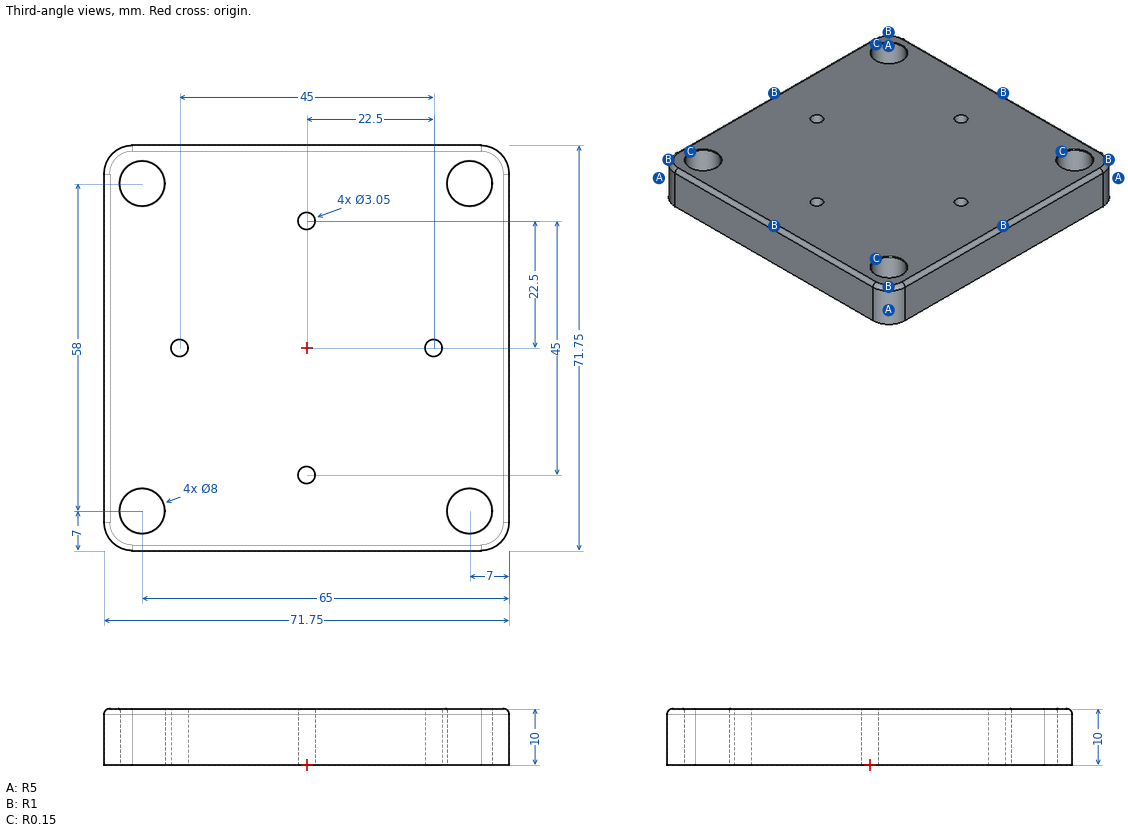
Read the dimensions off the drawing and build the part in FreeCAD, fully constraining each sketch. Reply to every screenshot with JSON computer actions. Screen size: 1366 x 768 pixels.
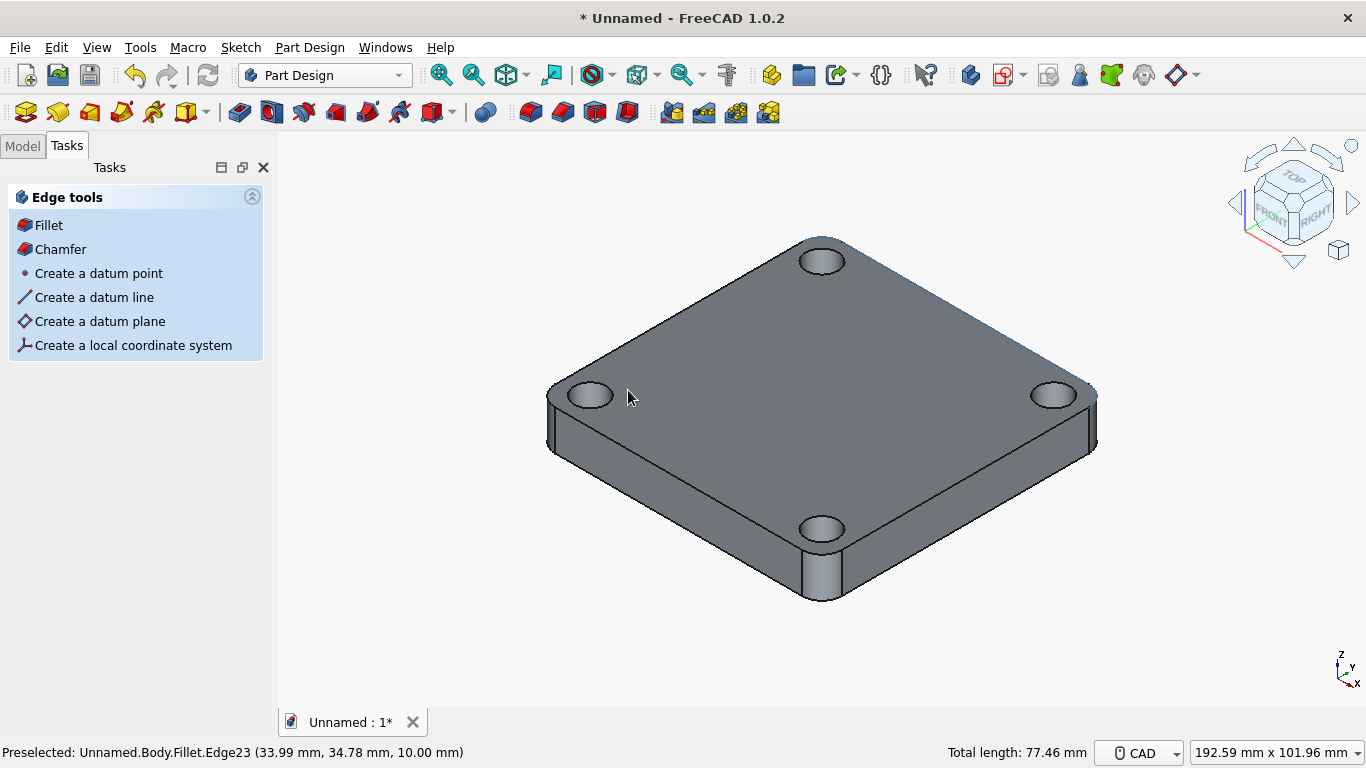
{"action": "left_click", "coordinate": [965, 478], "text": "ctrl"}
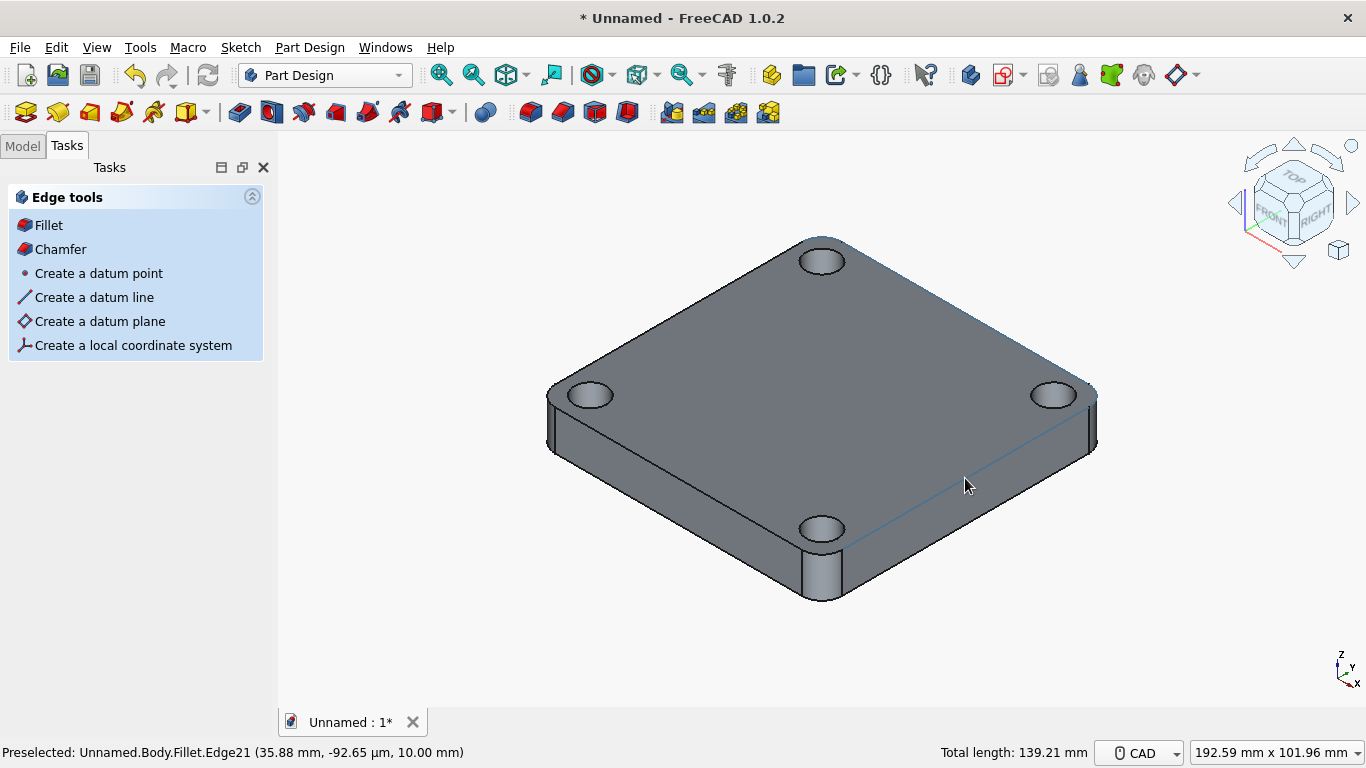
{"action": "left_click", "coordinate": [679, 478], "text": "ctrl"}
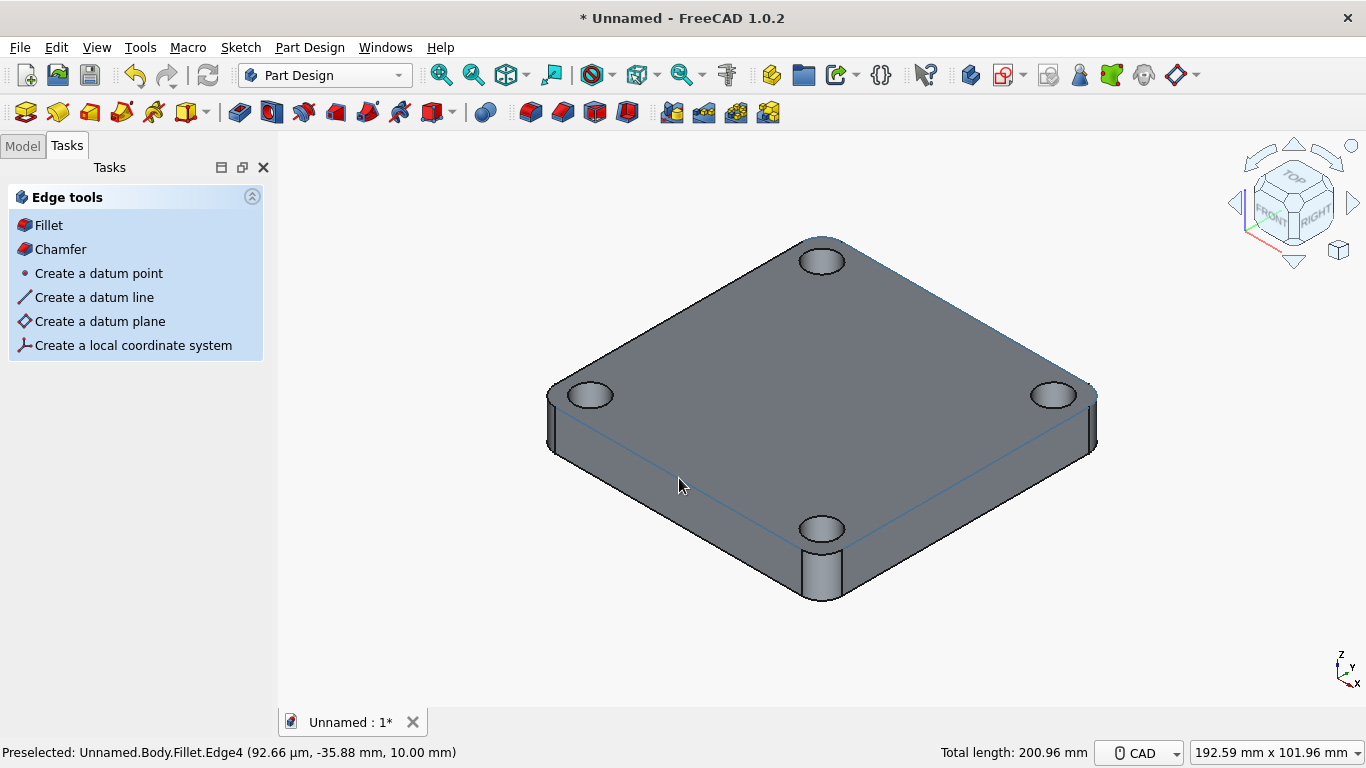
{"action": "left_click", "coordinate": [547, 395], "text": "ctrl"}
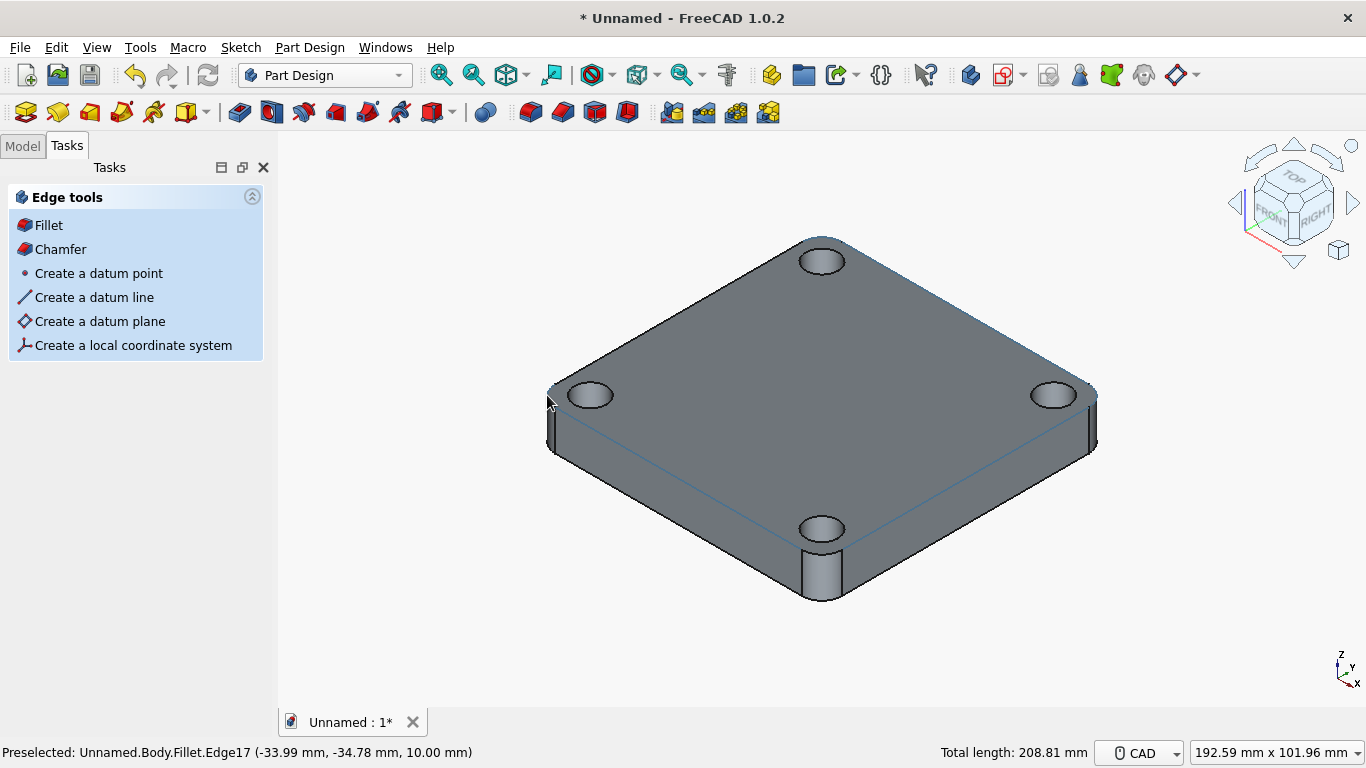
{"action": "left_click", "coordinate": [822, 554], "text": "ctrl"}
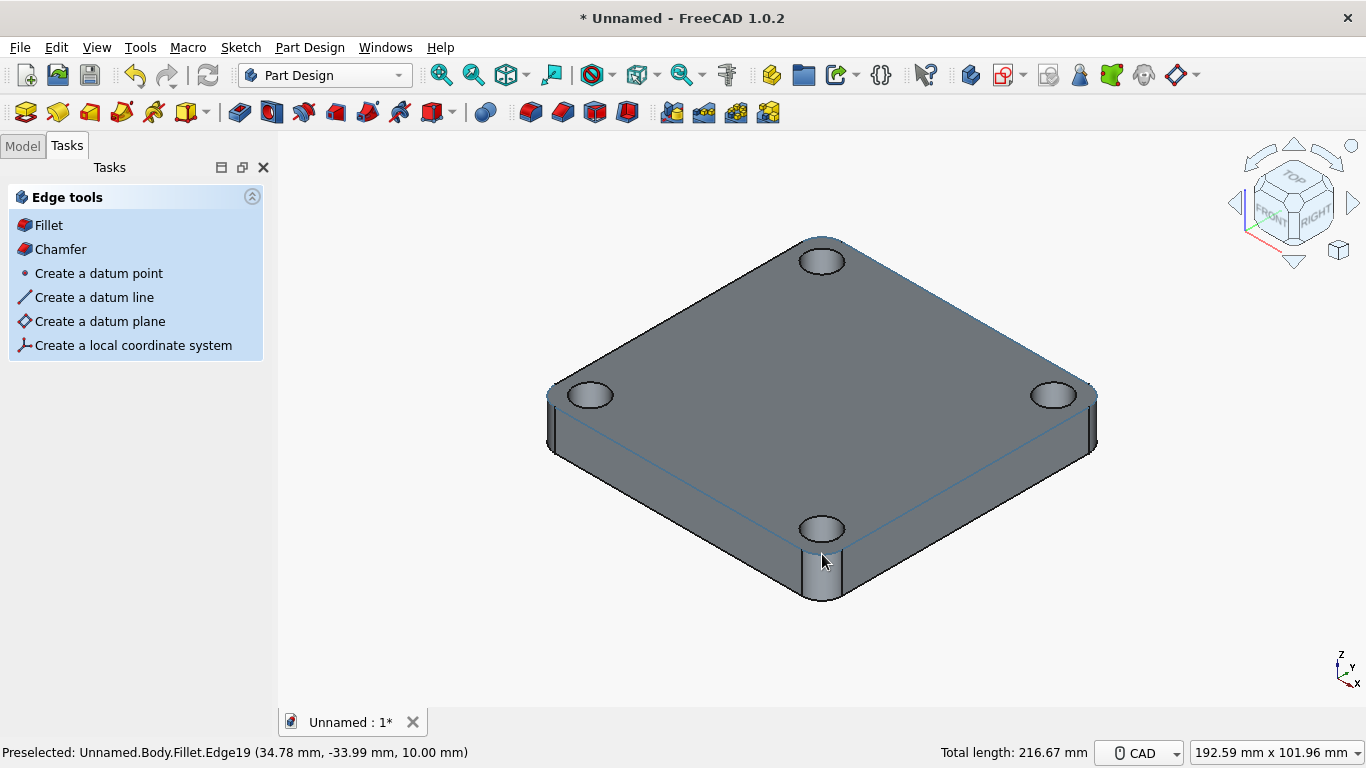
{"action": "key", "text": "2"}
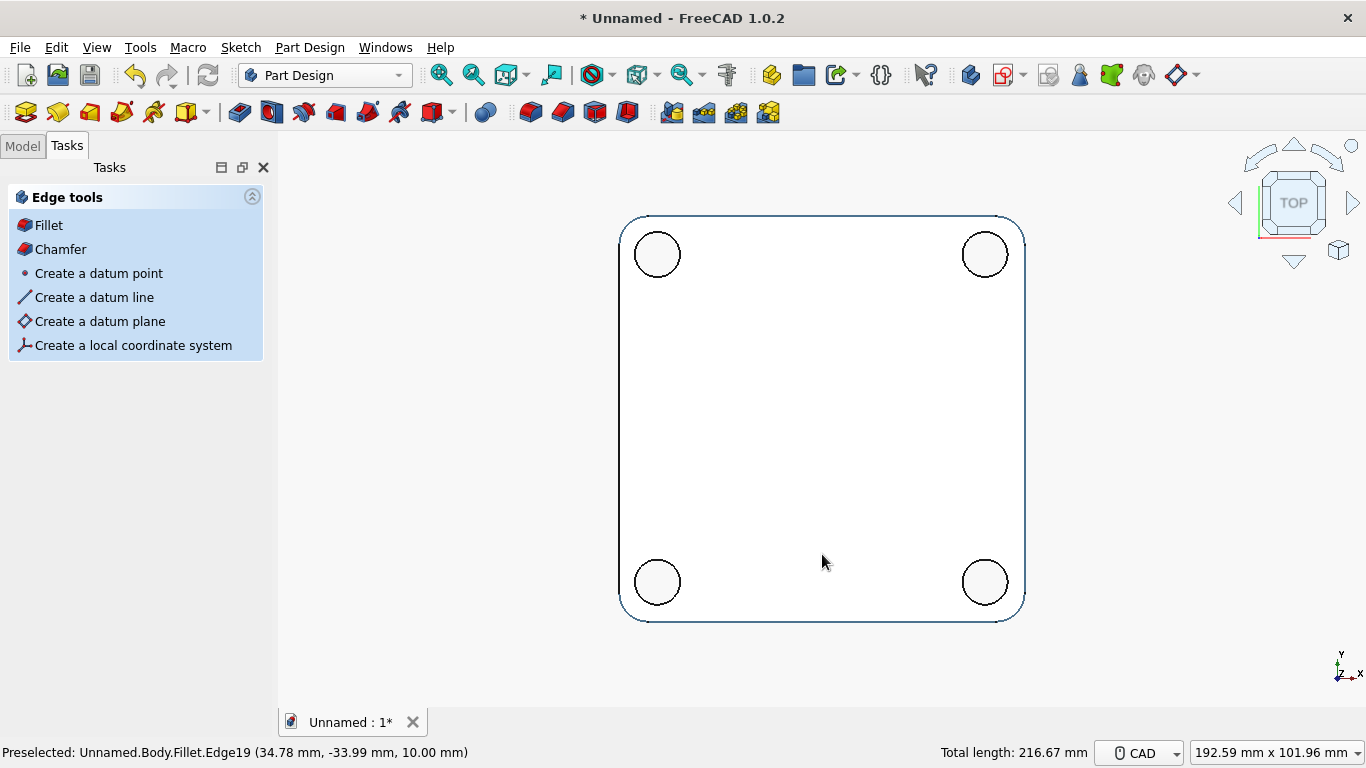
{"action": "left_click", "coordinate": [619, 418], "text": "ctrl"}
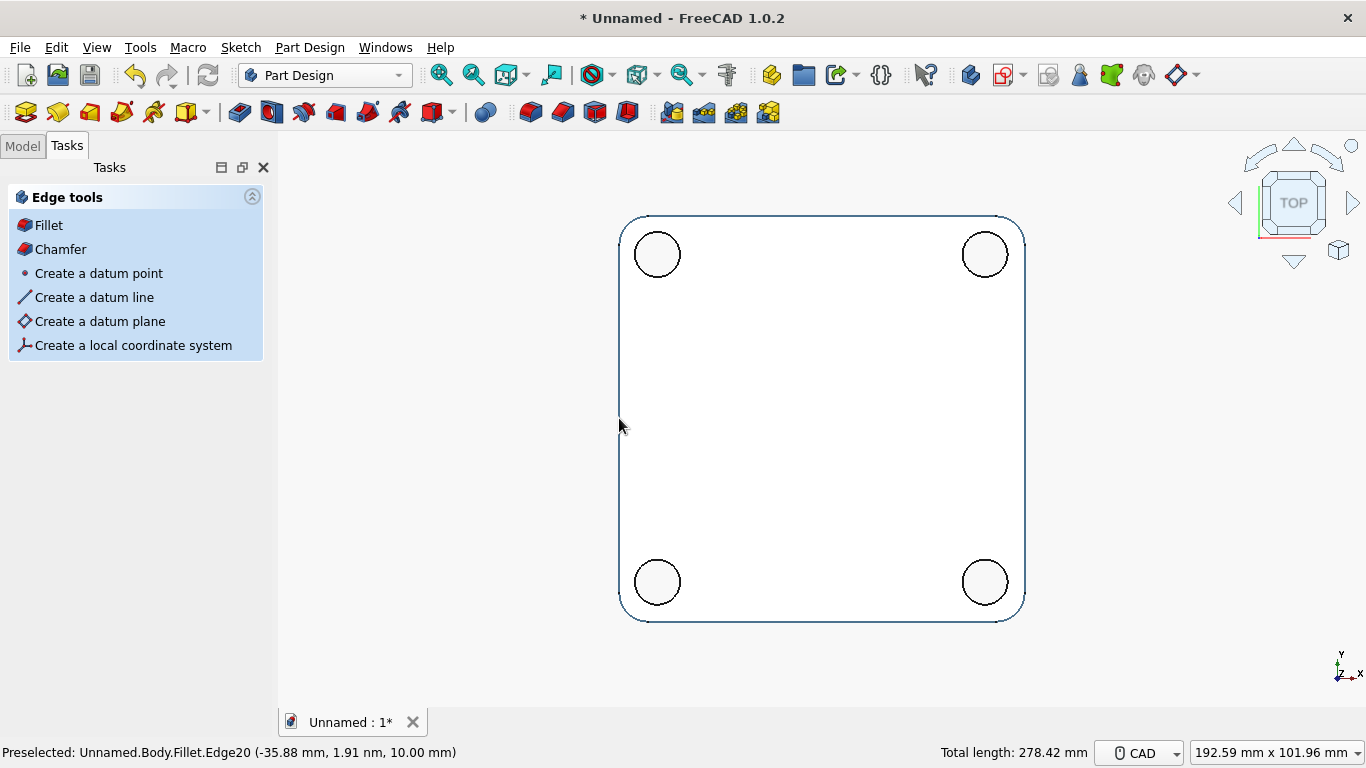
{"action": "left_click", "coordinate": [532, 112]}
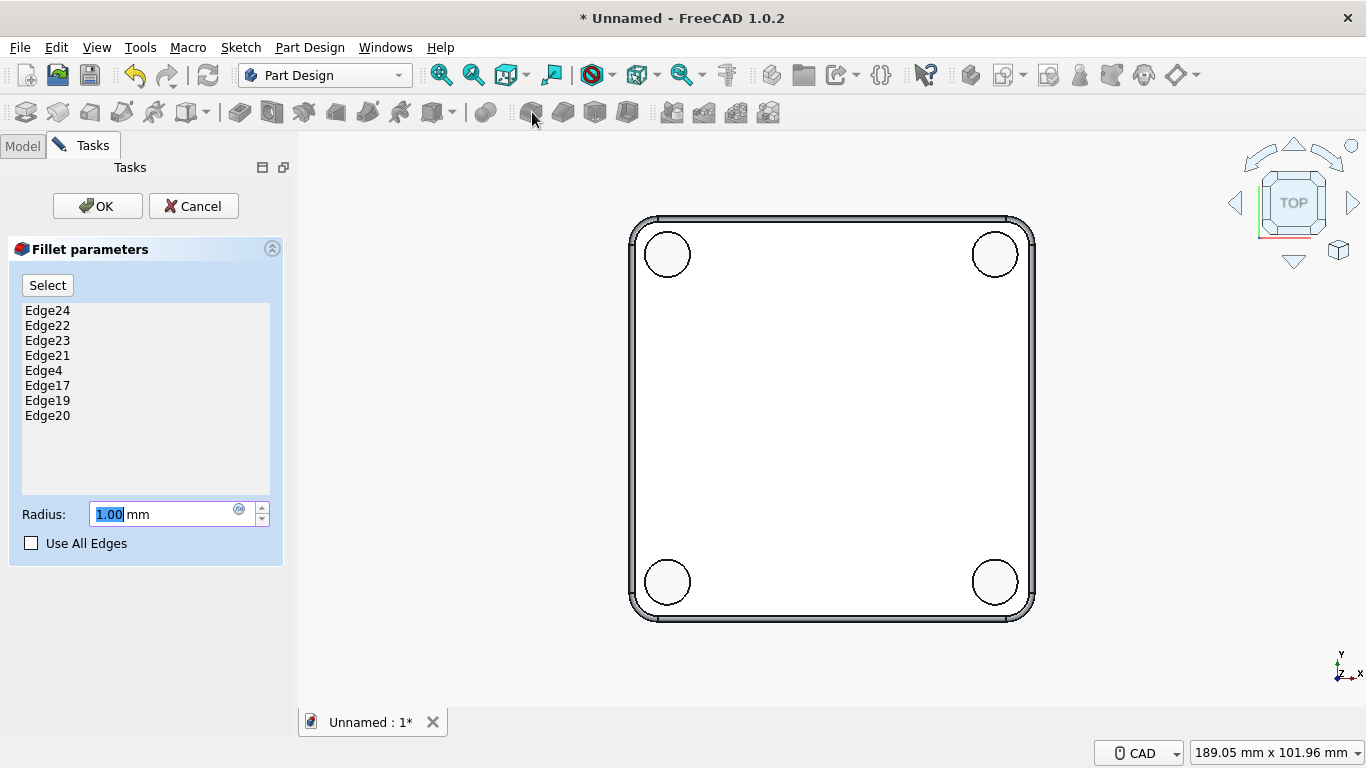
{"action": "type", "text": "1"}
{"action": "key", "text": "Tab"}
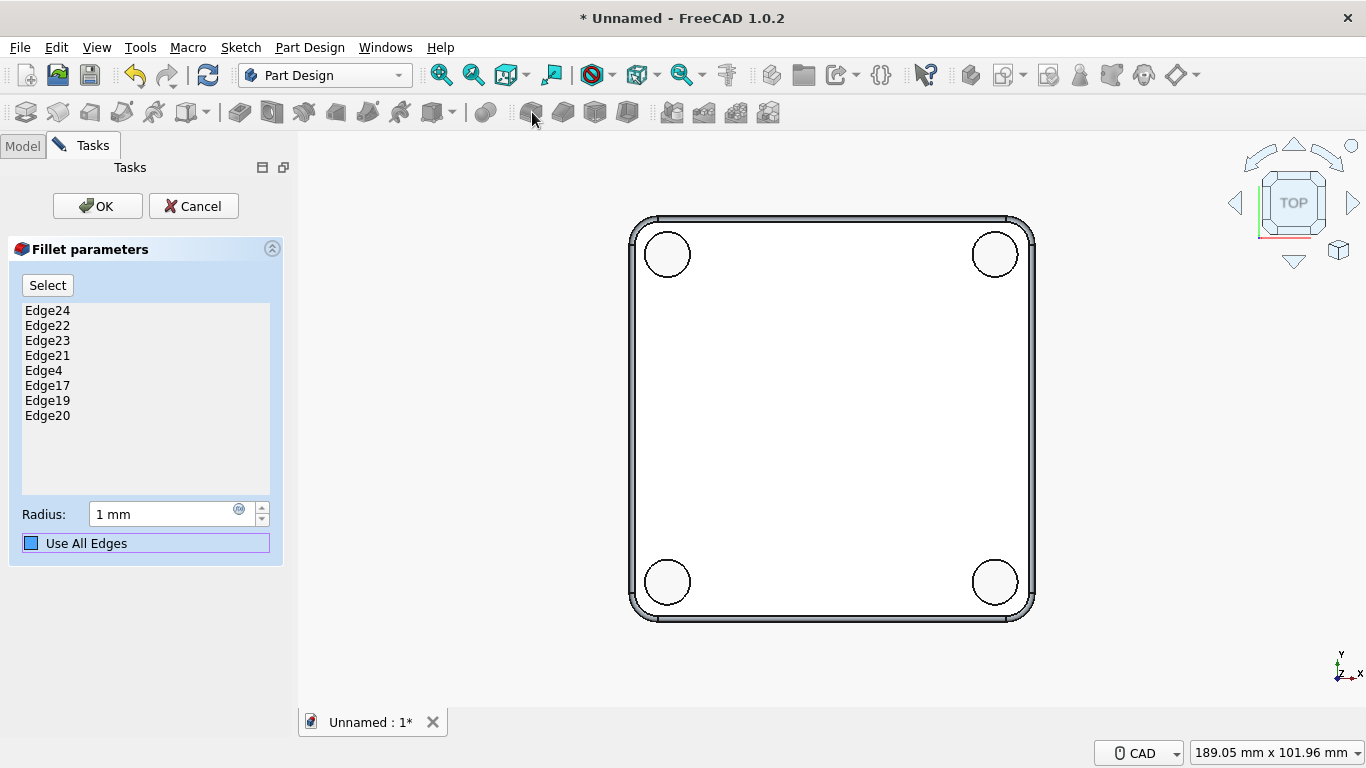
{"action": "left_click", "coordinate": [98, 206]}